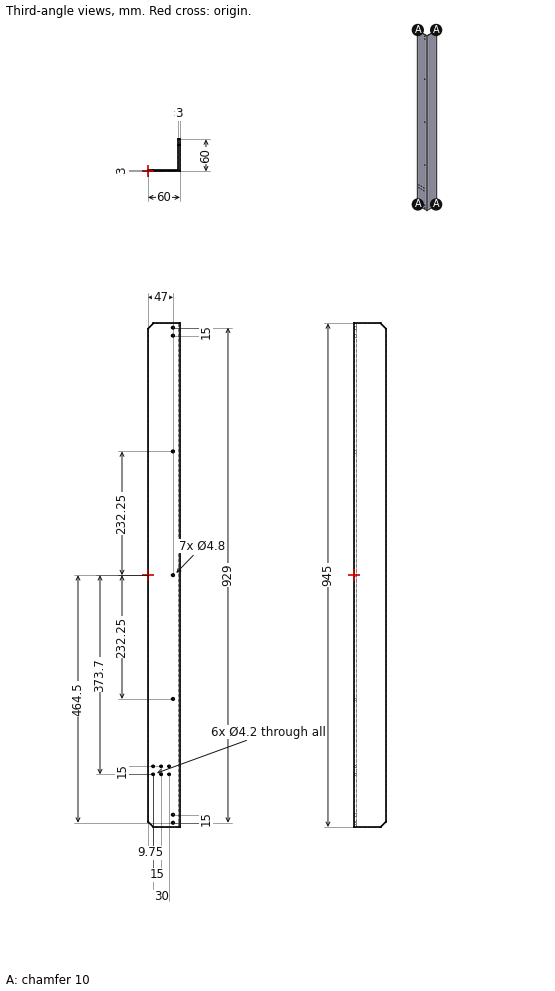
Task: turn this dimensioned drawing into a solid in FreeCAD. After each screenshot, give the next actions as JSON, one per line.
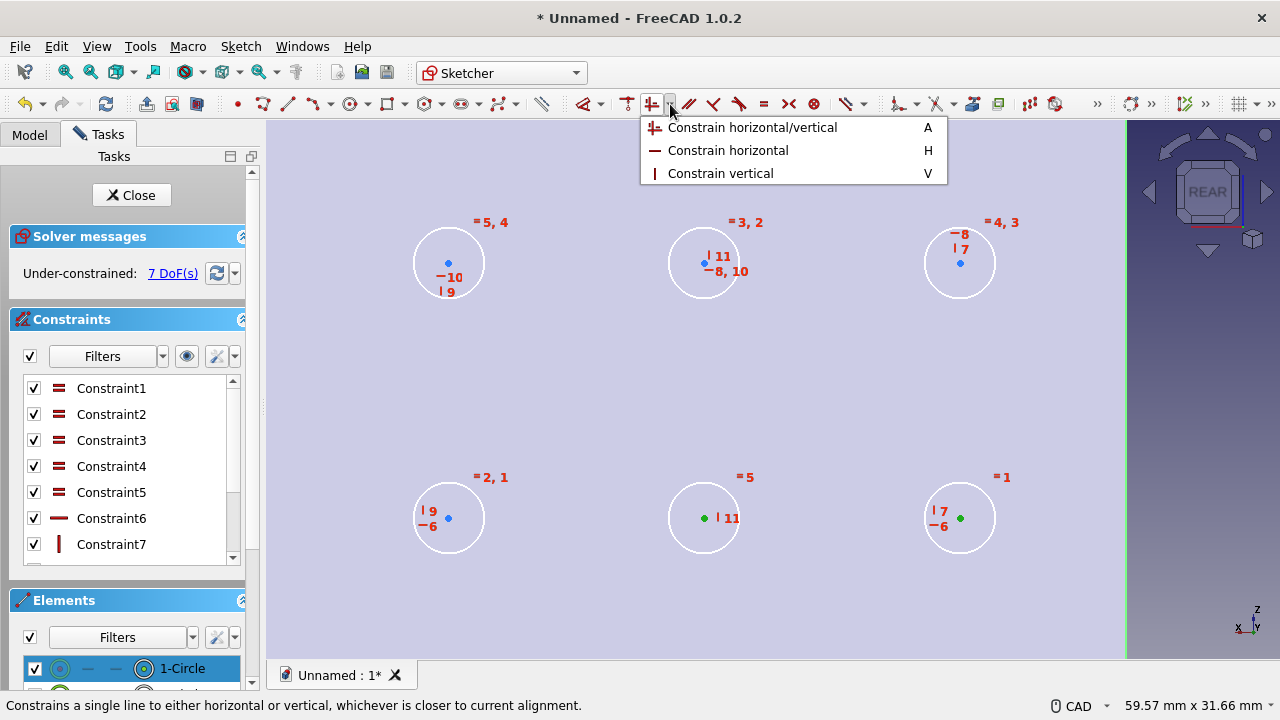
{"action": "left_click", "coordinate": [794, 150]}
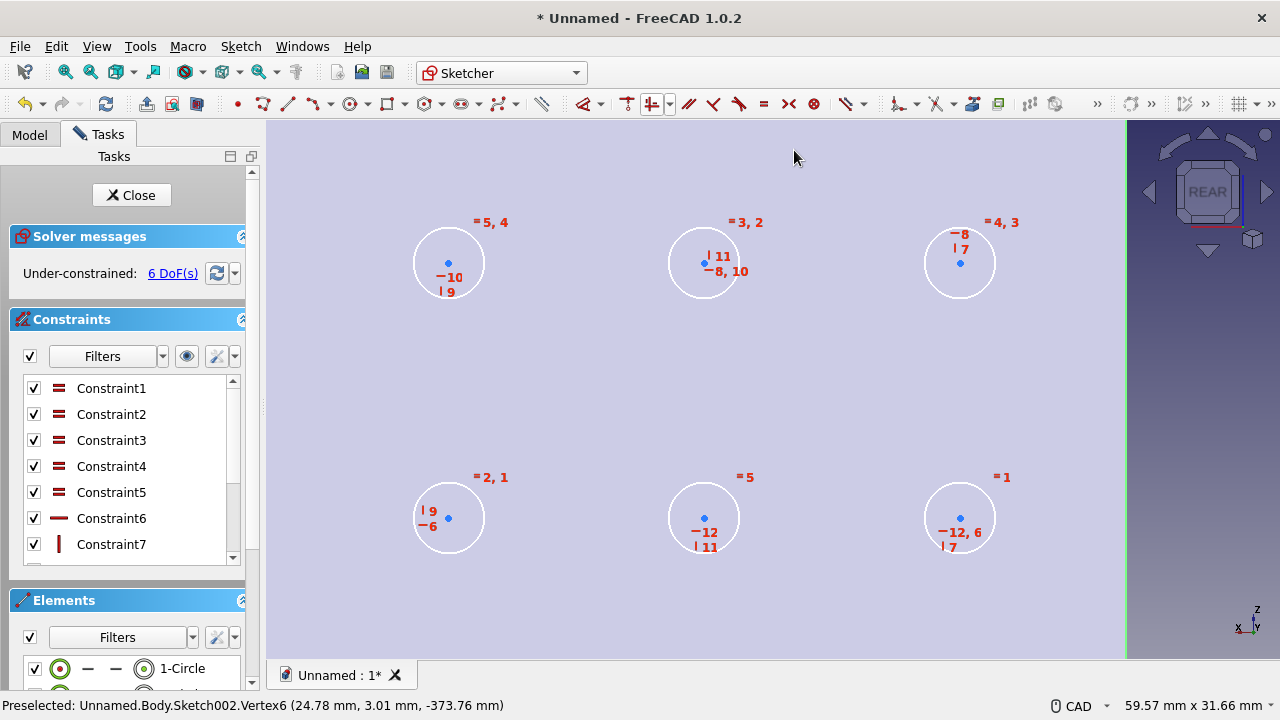
{"action": "left_click", "coordinate": [582, 104]}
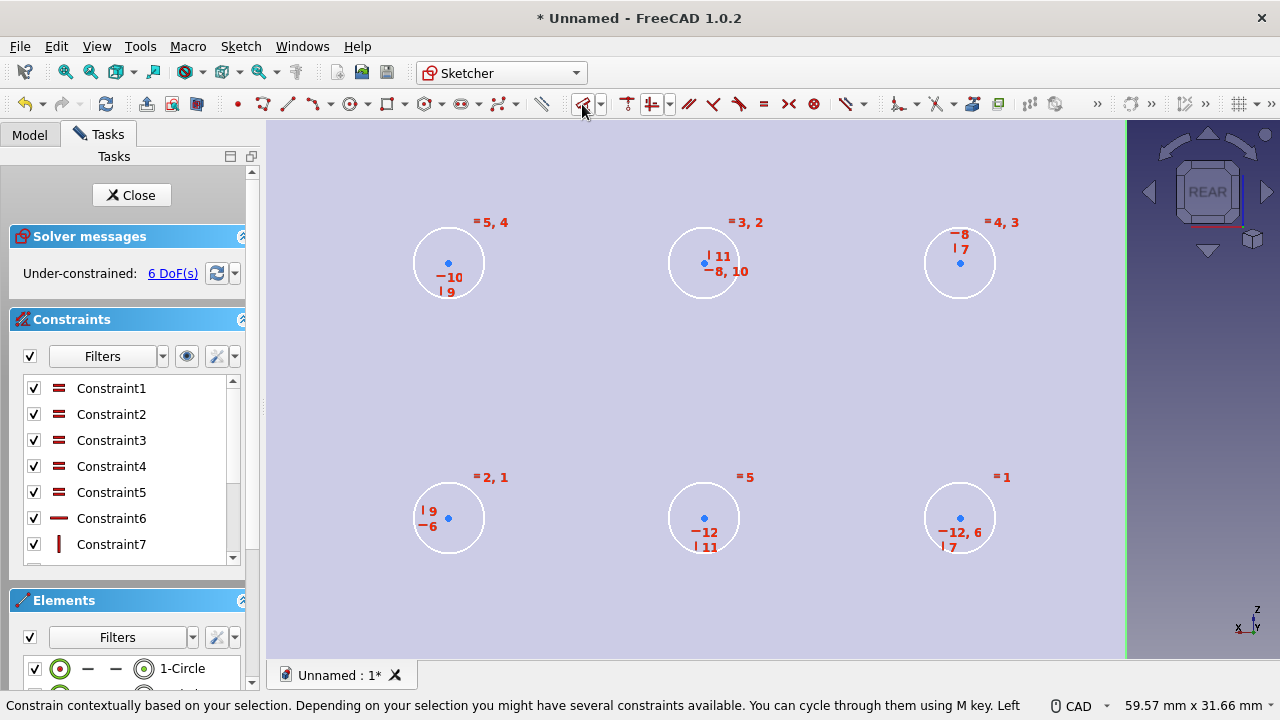
{"action": "left_click", "coordinate": [985, 493]}
{"action": "left_click", "coordinate": [1008, 470]}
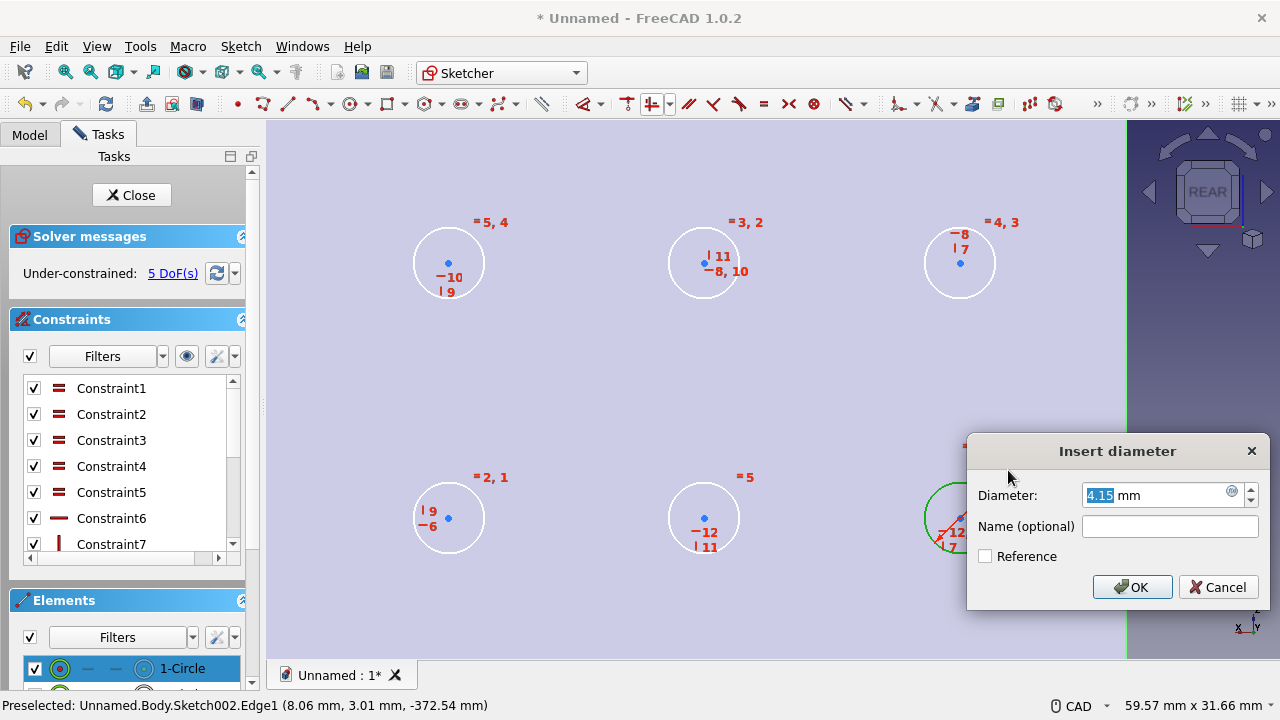
{"action": "type", "text": "4.2"}
{"action": "key", "text": "Return"}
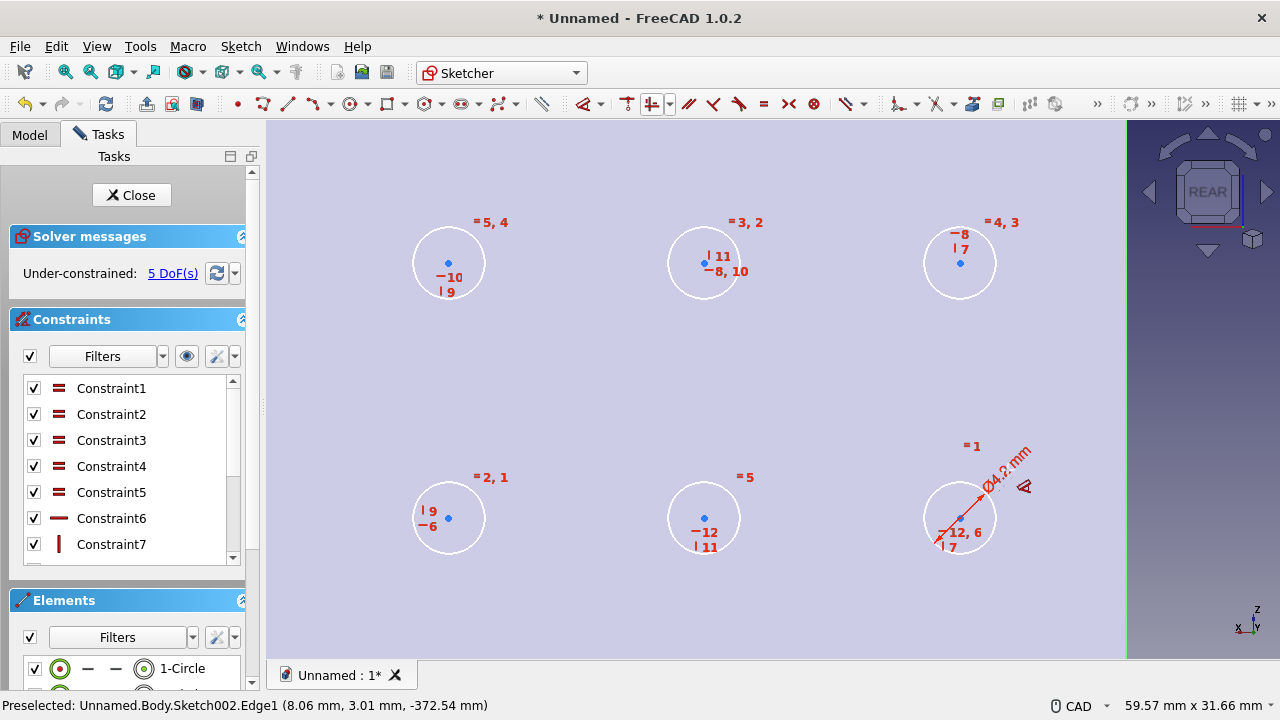
{"action": "left_click", "coordinate": [960, 518]}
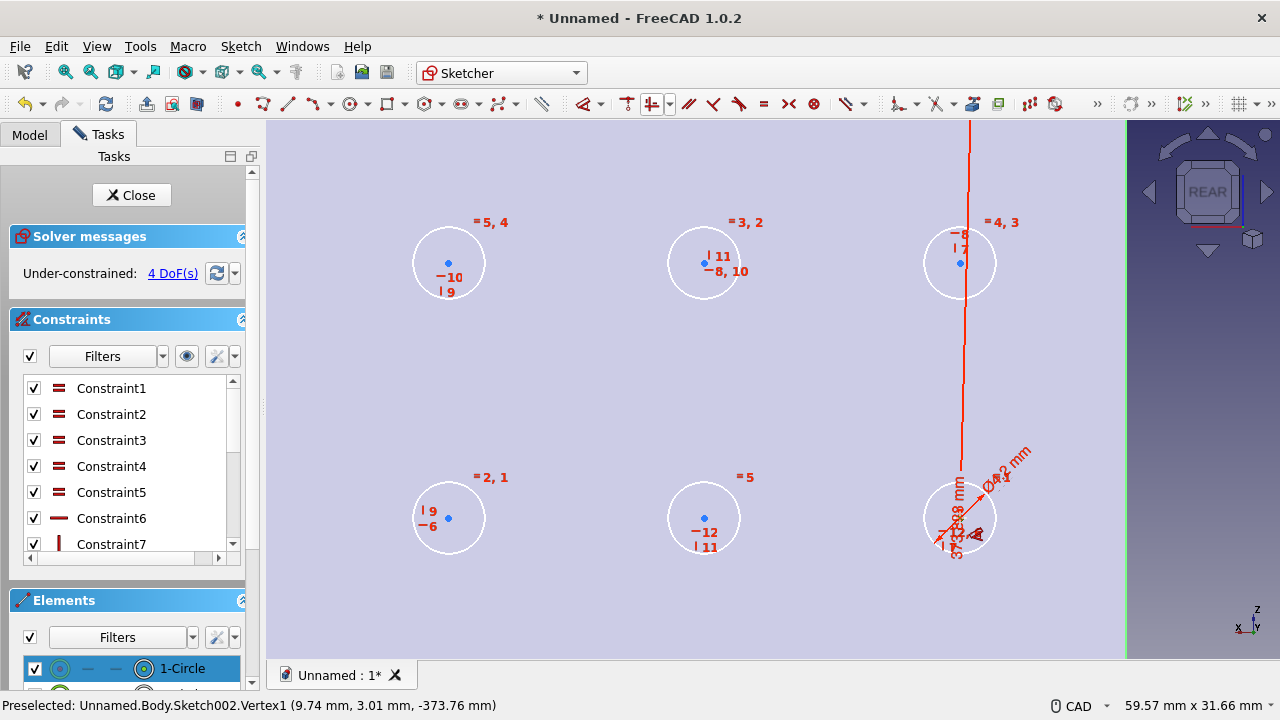
{"action": "left_click", "coordinate": [449, 518]}
{"action": "left_click", "coordinate": [587, 552]}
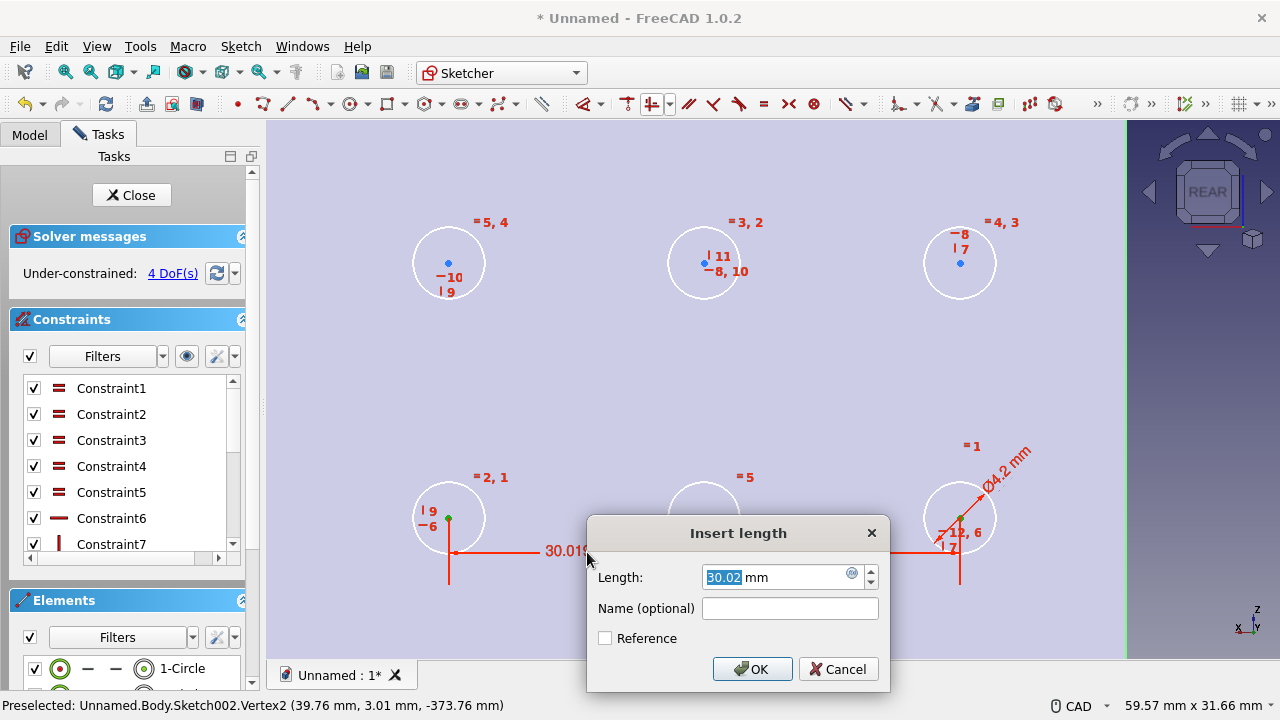
{"action": "type", "text": "30"}
{"action": "key", "text": "Return"}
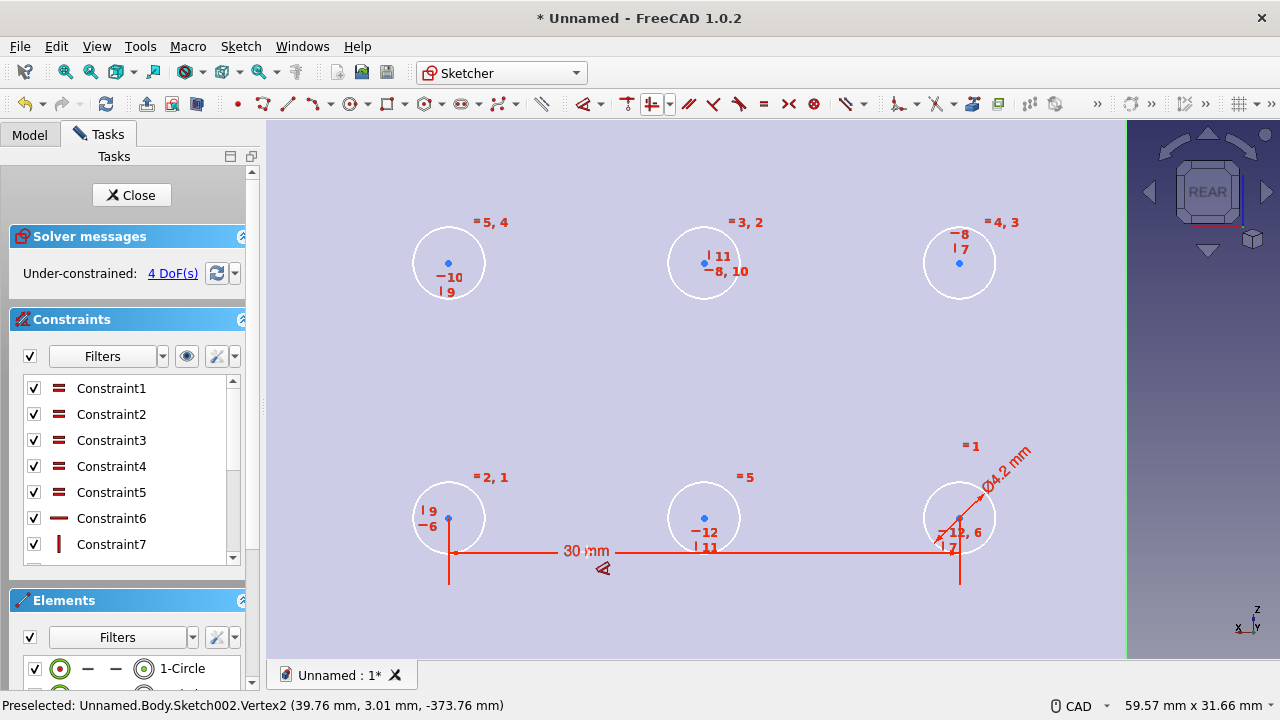
{"action": "left_click", "coordinate": [960, 518]}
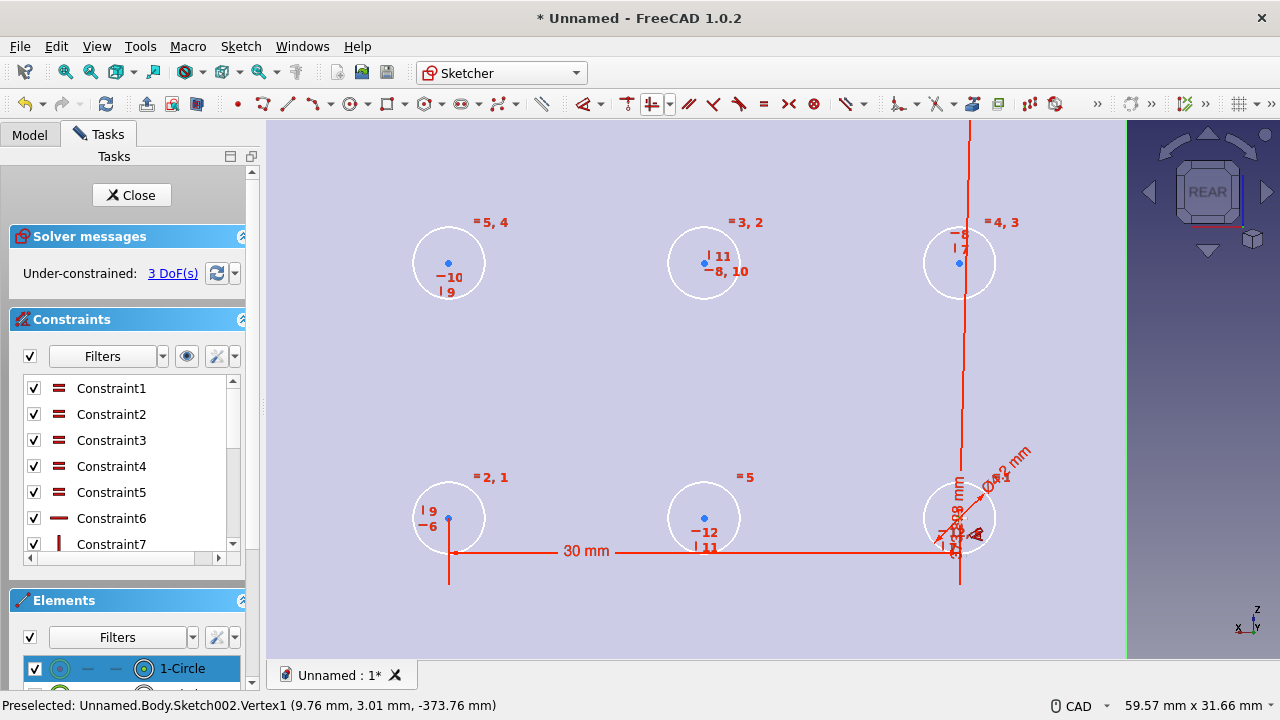
{"action": "left_click", "coordinate": [704, 263]}
{"action": "left_click", "coordinate": [832, 552]}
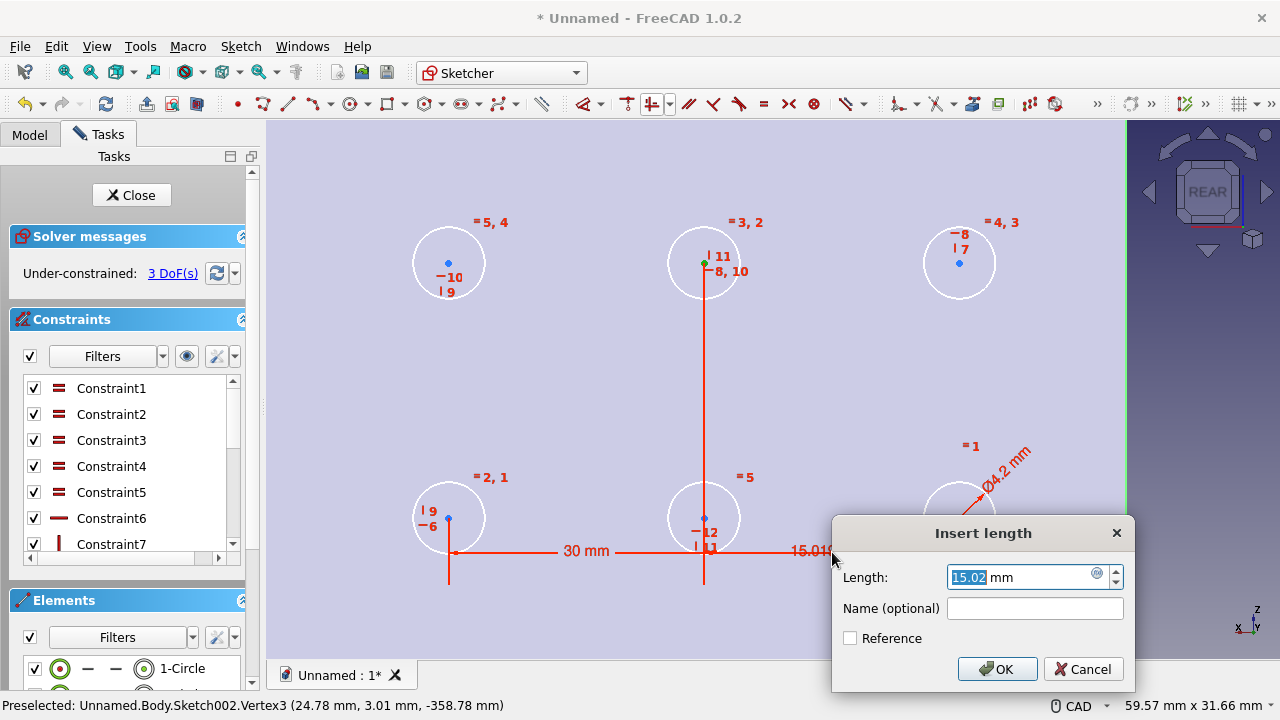
{"action": "type", "text": "15"}
{"action": "key", "text": "Return"}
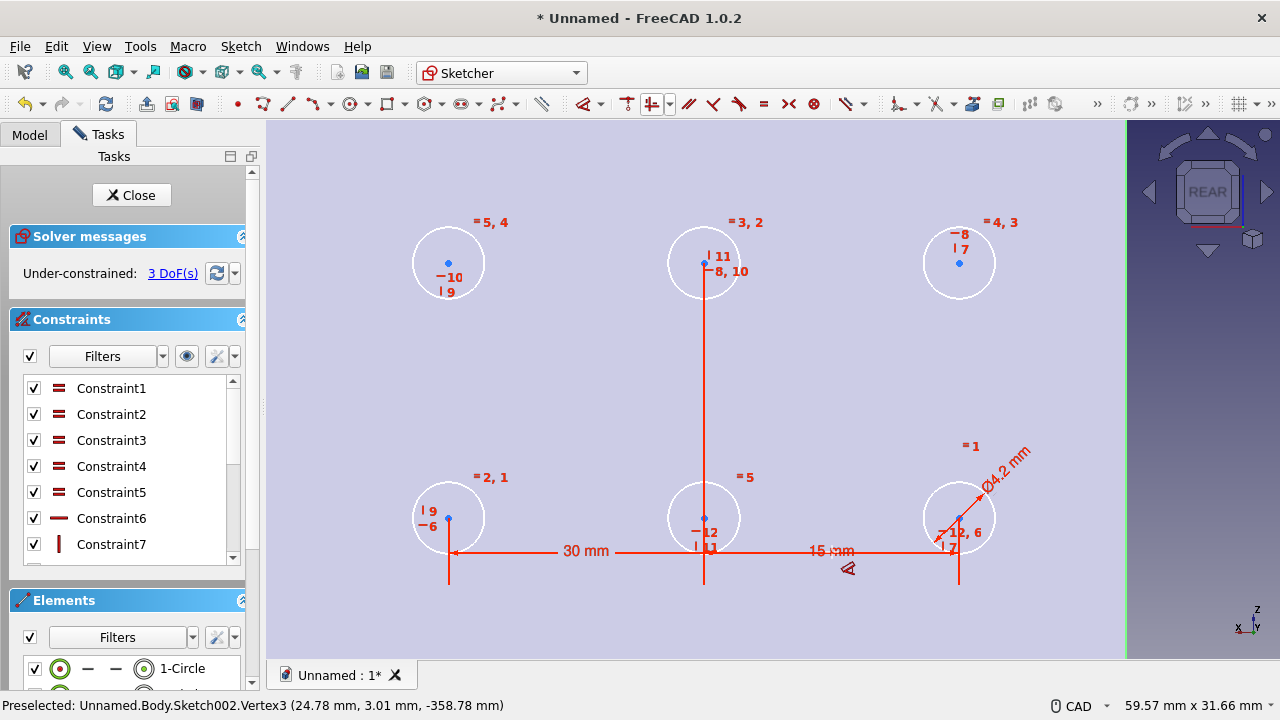
{"action": "left_click", "coordinate": [959, 518]}